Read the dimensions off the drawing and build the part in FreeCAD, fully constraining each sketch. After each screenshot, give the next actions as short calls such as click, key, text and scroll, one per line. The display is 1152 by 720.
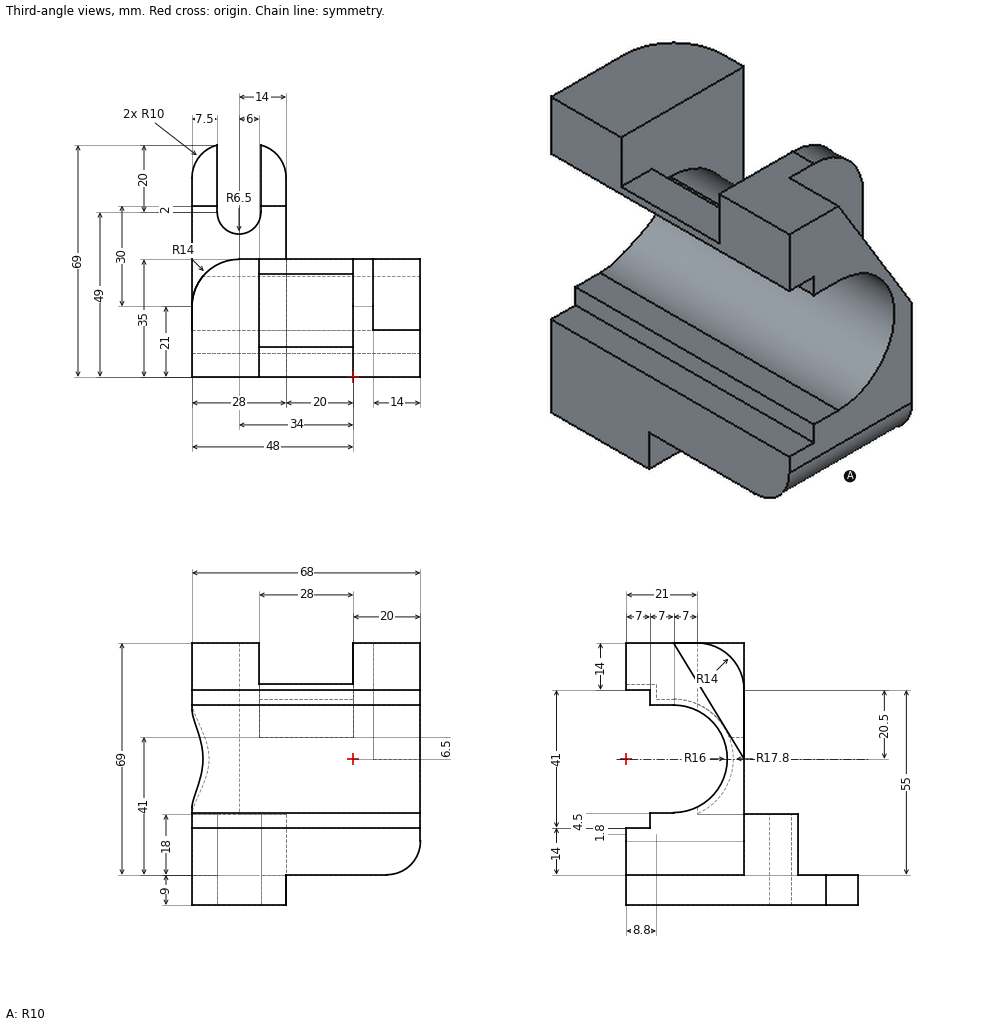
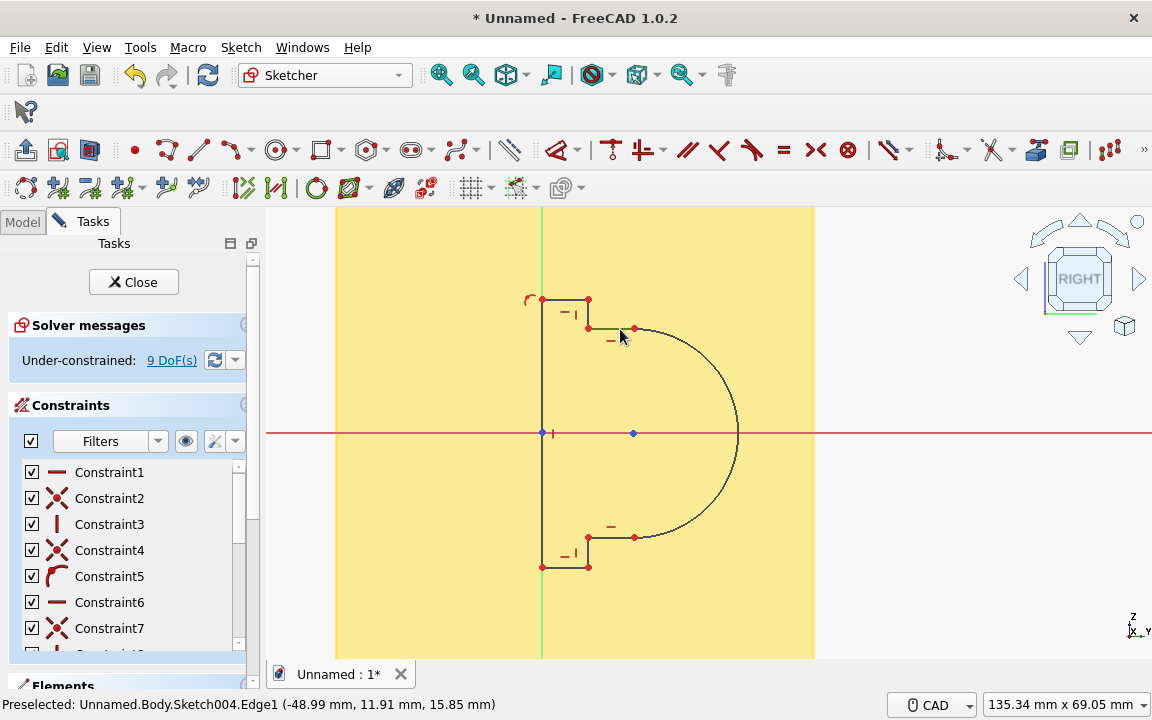
click(718, 495)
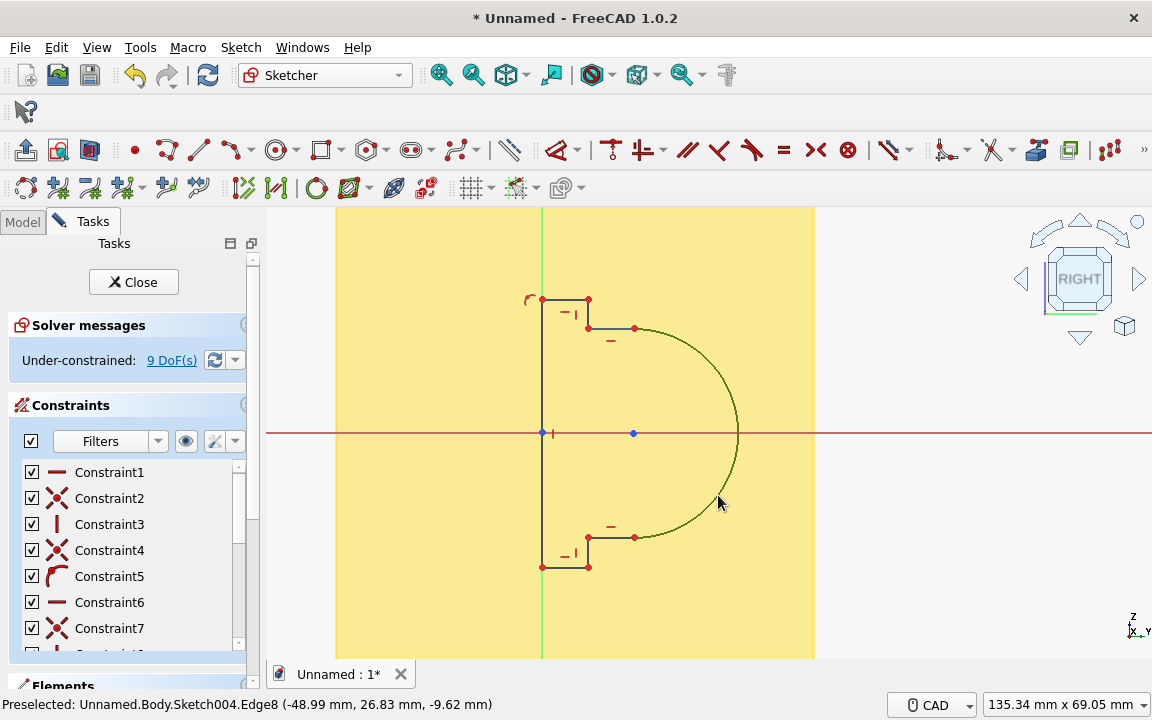
click(752, 150)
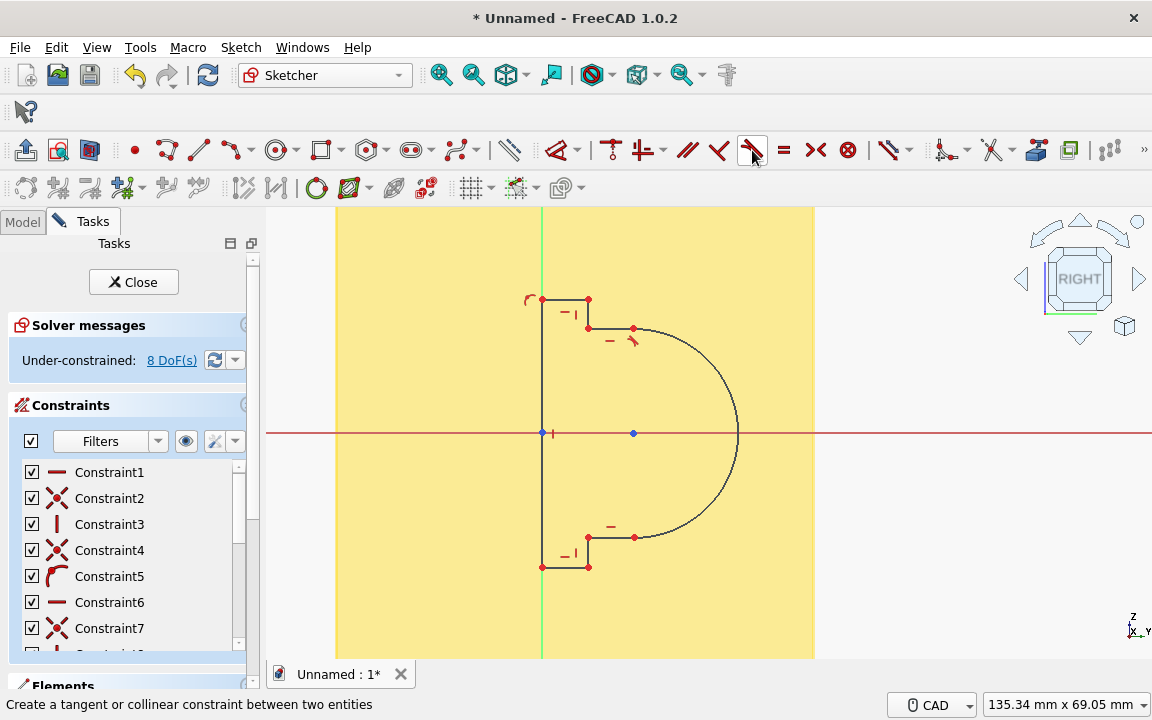
click(602, 538)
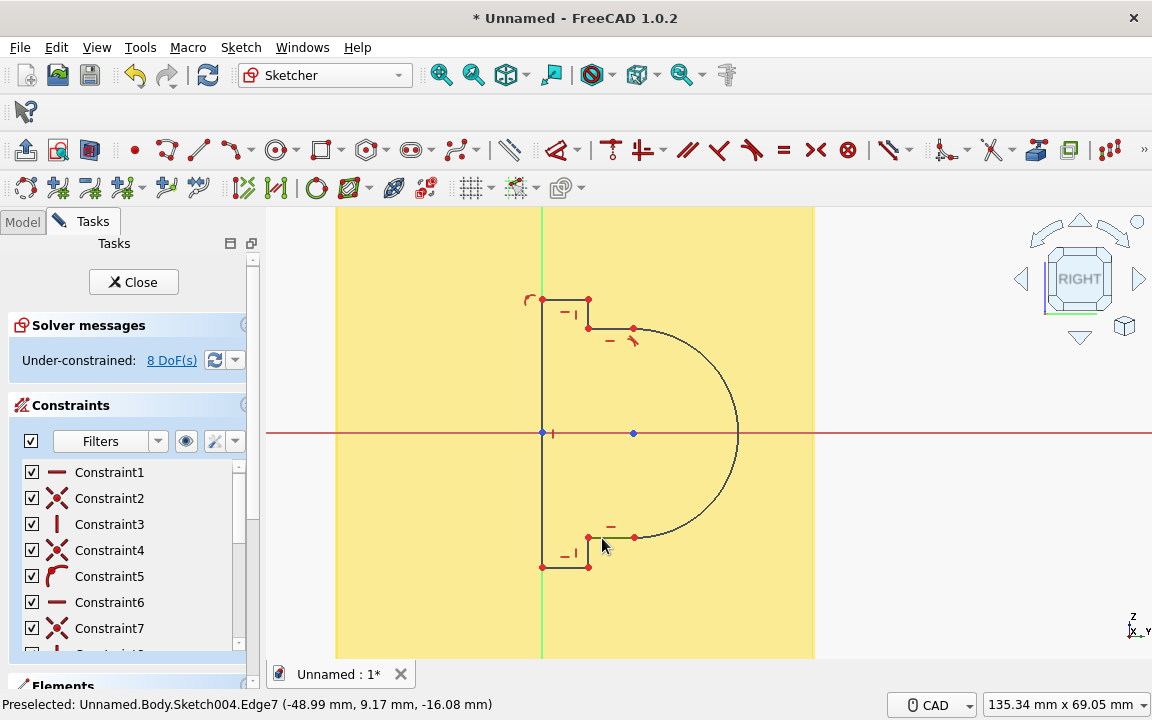
click(718, 495)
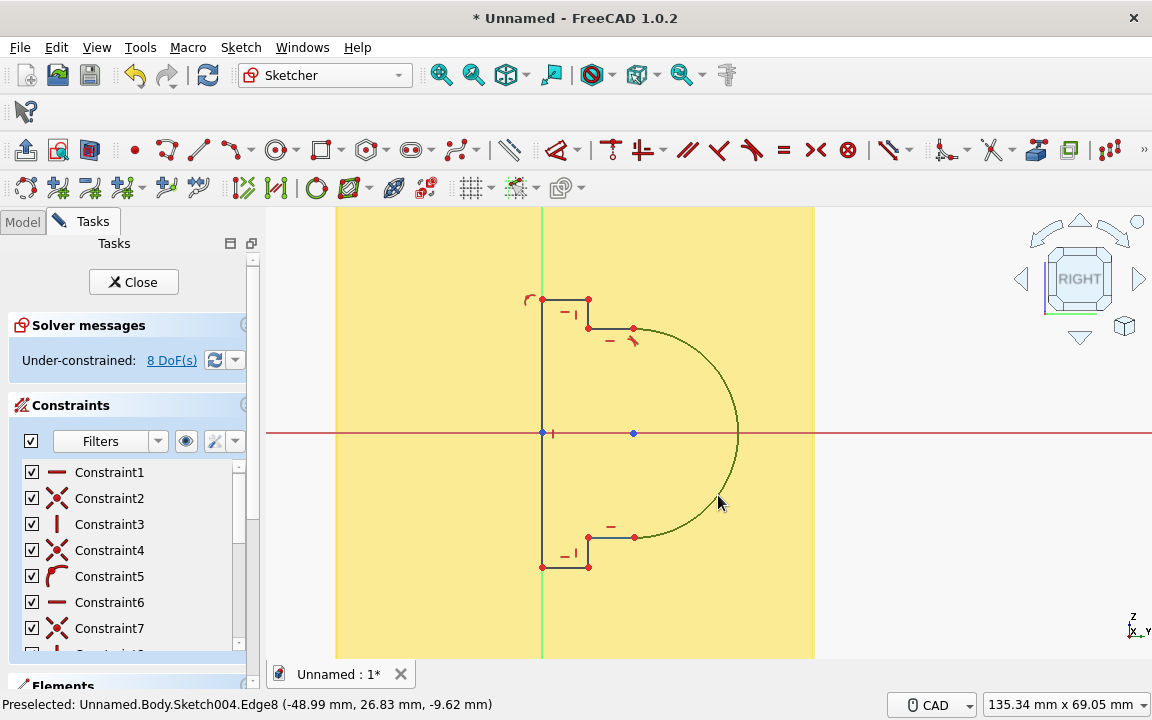
key(t)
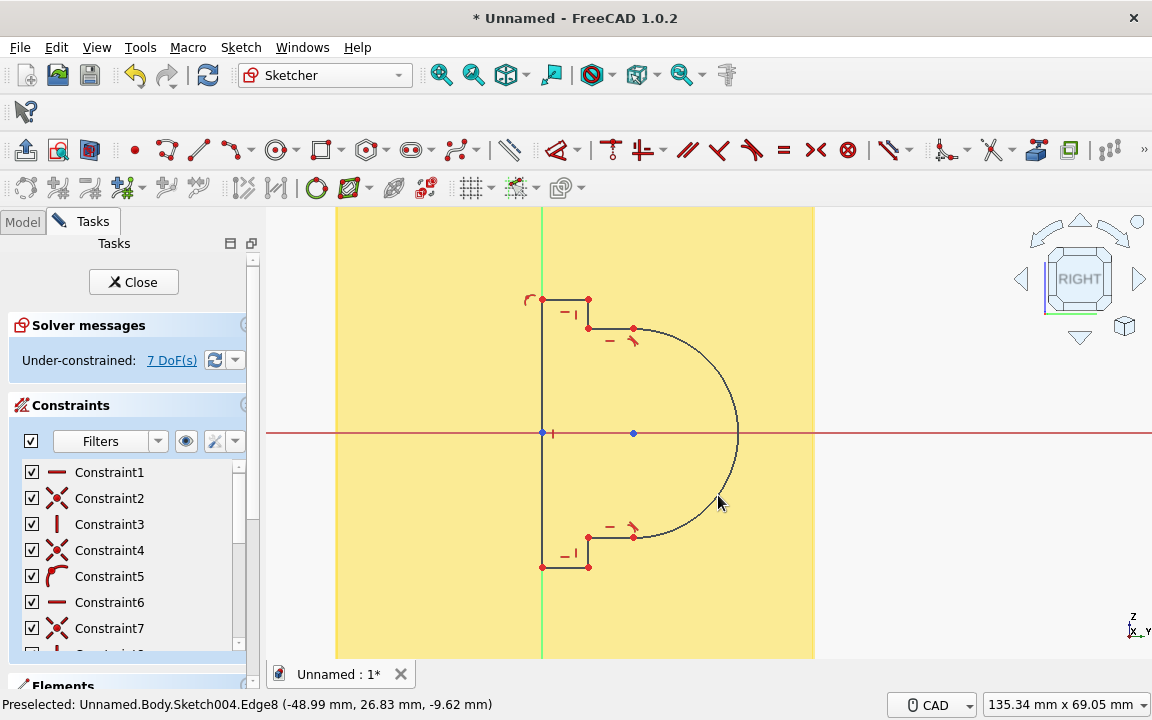
click(634, 433)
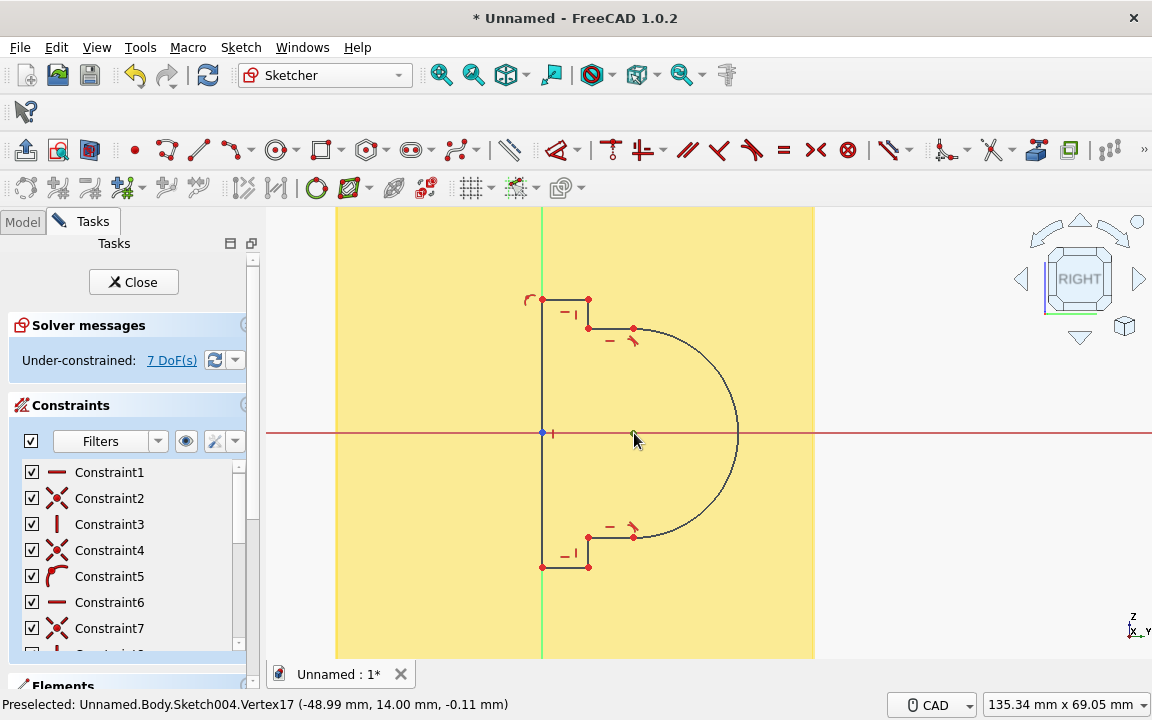
click(344, 433)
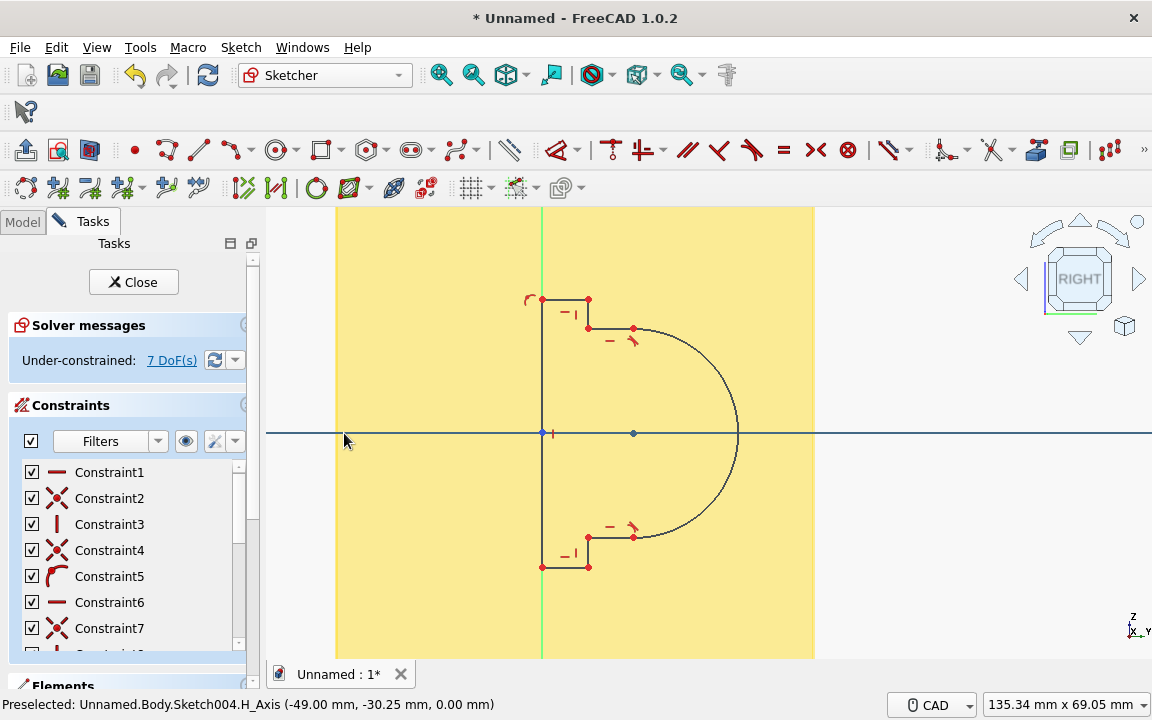
click(612, 150)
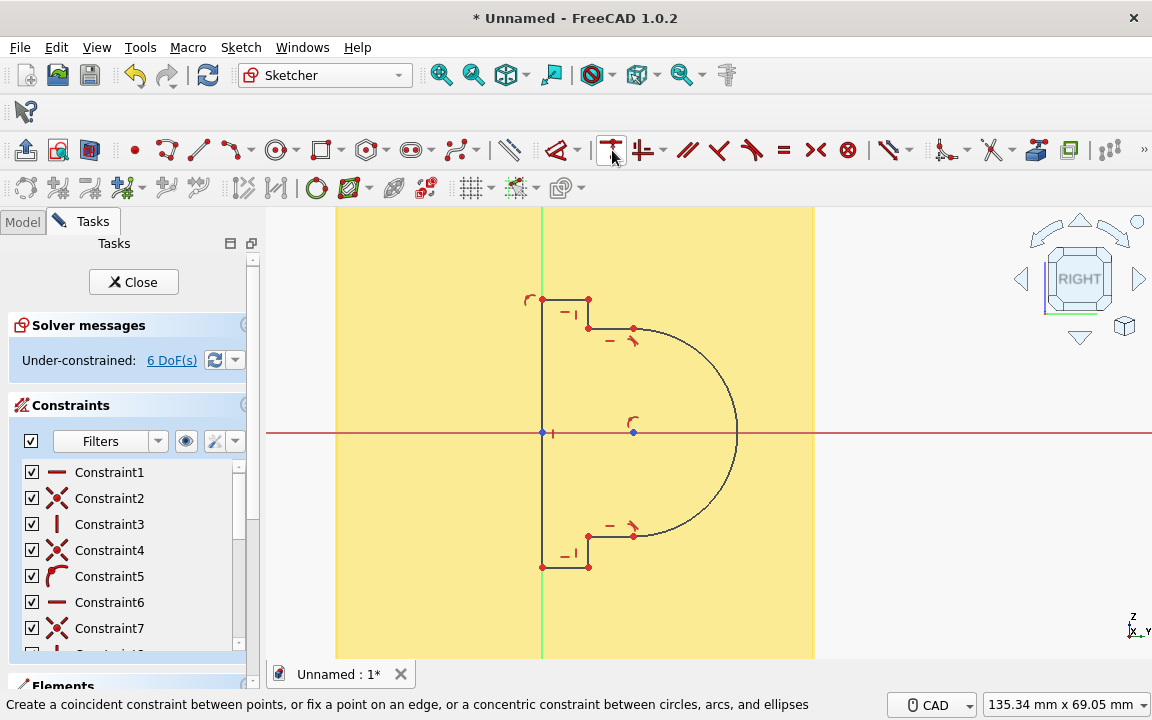
click(588, 300)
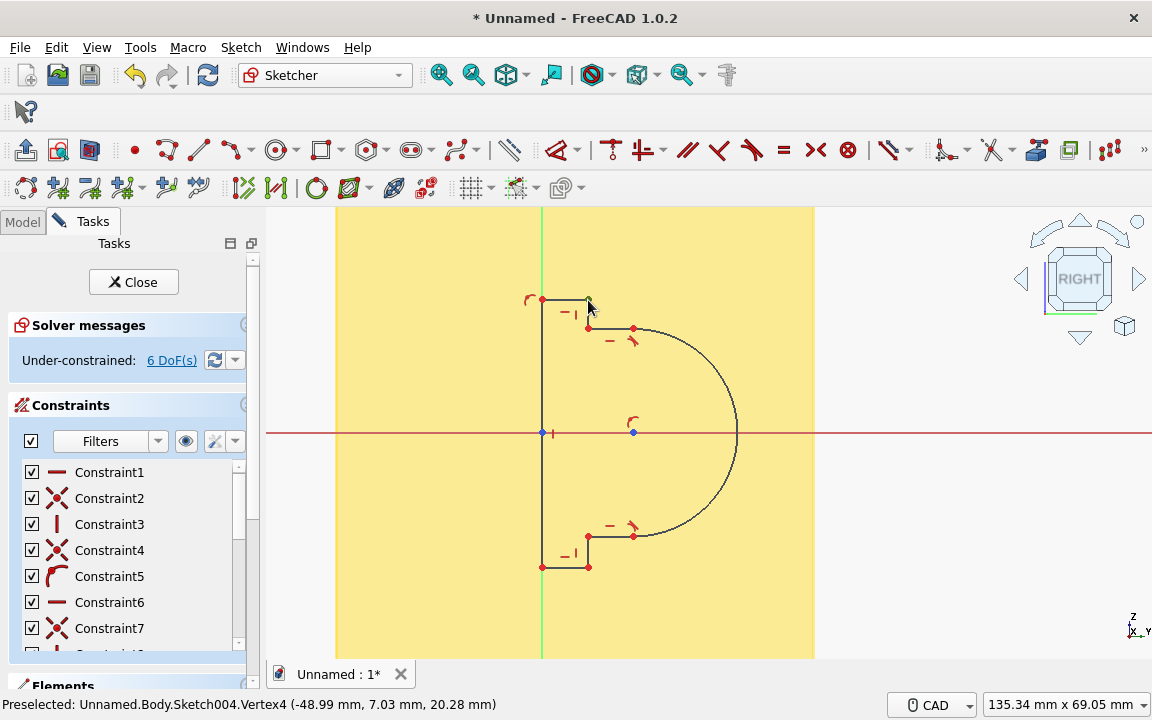
click(588, 568)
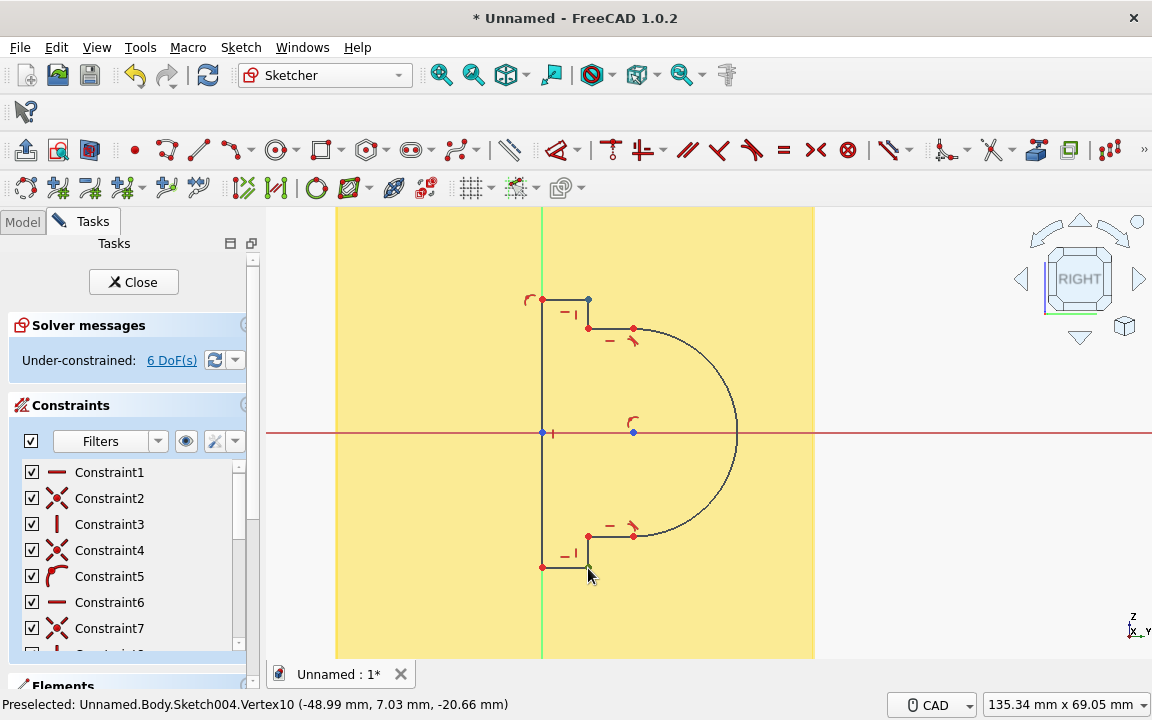
click(344, 433)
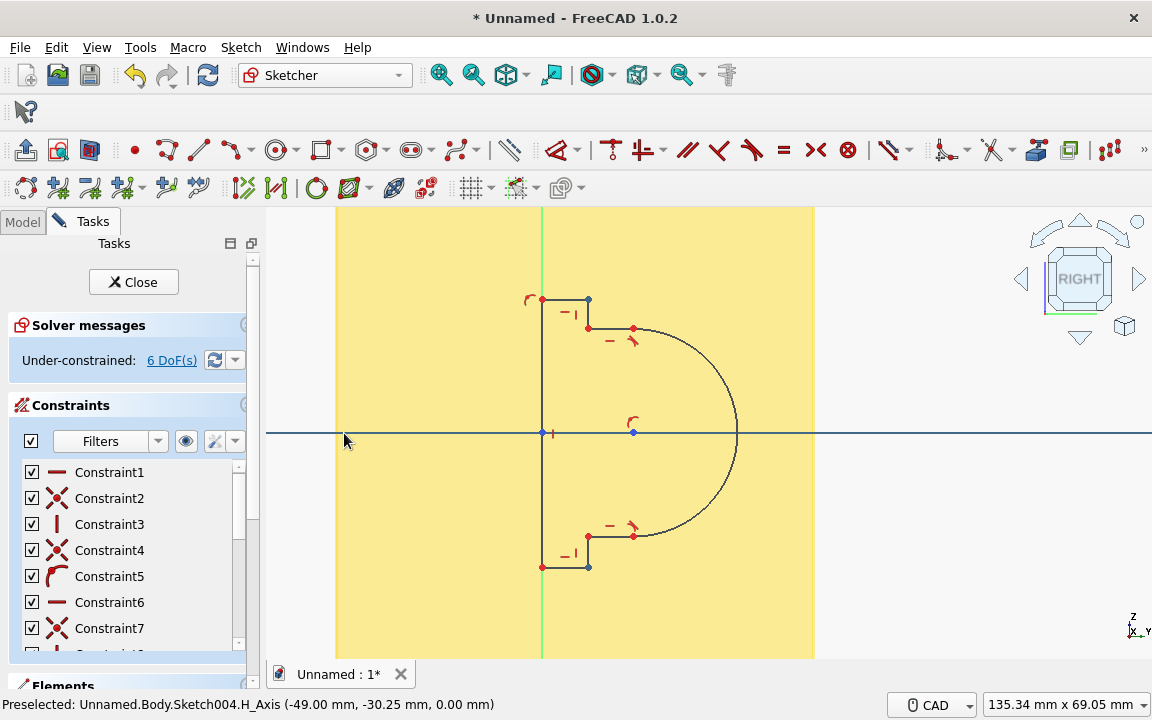
key(s)